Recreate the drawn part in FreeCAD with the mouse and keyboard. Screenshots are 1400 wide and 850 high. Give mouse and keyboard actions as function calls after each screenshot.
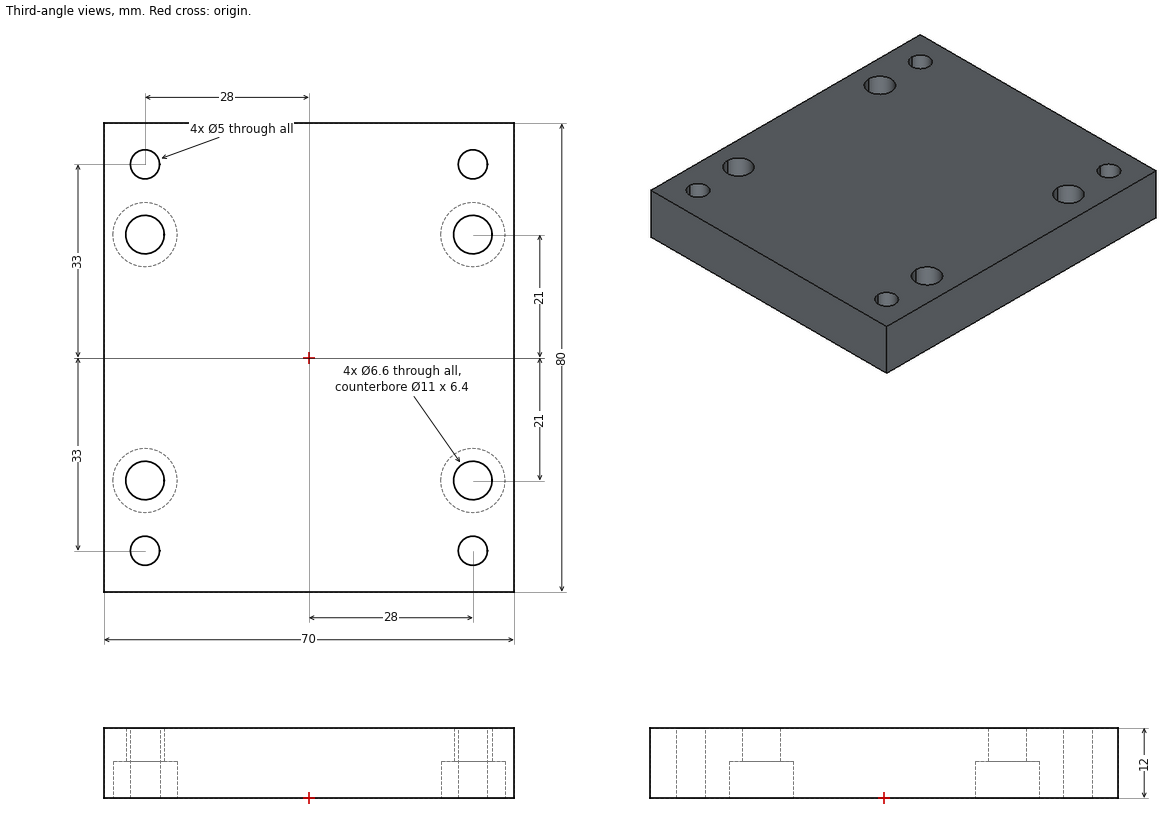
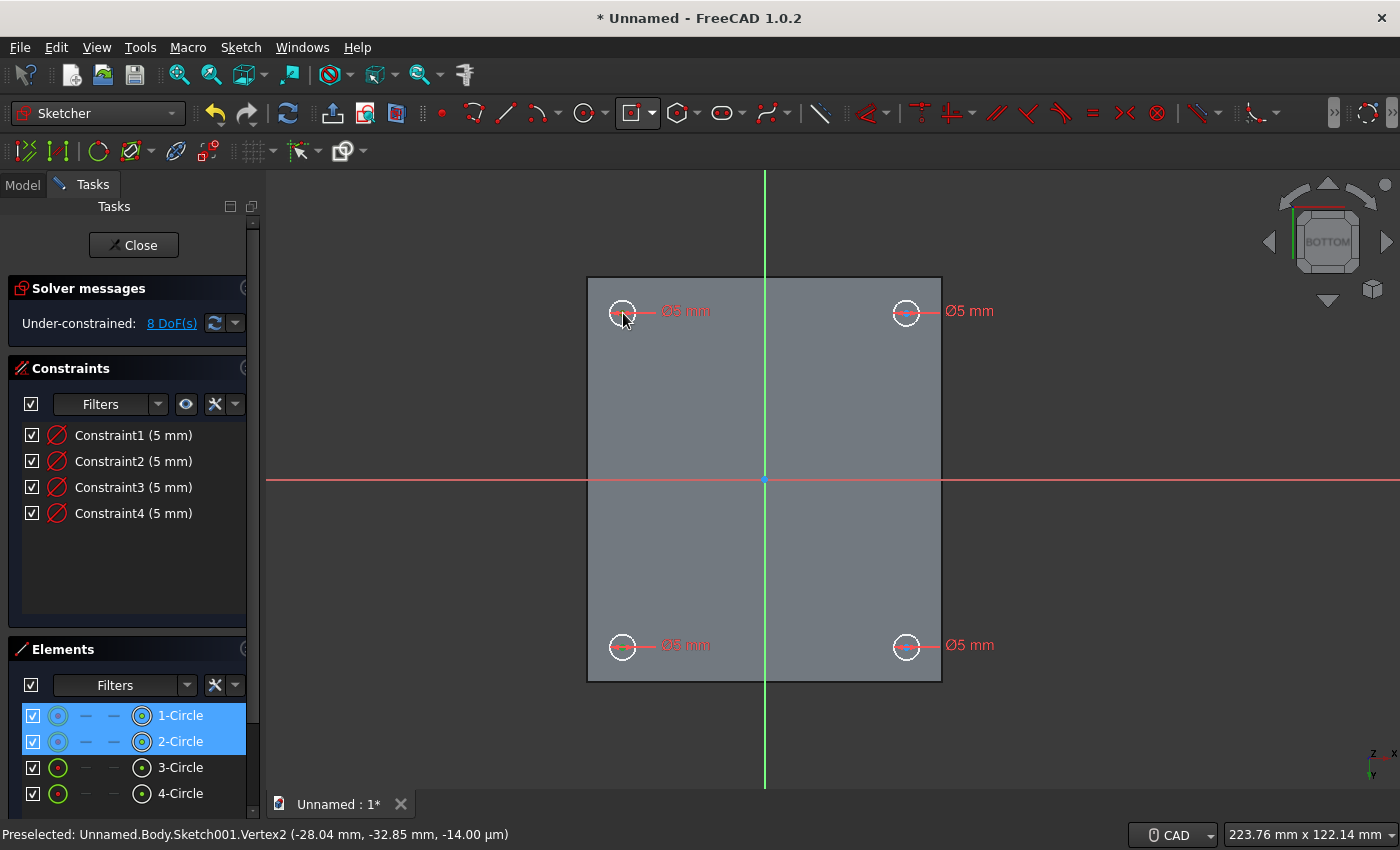
click(974, 114)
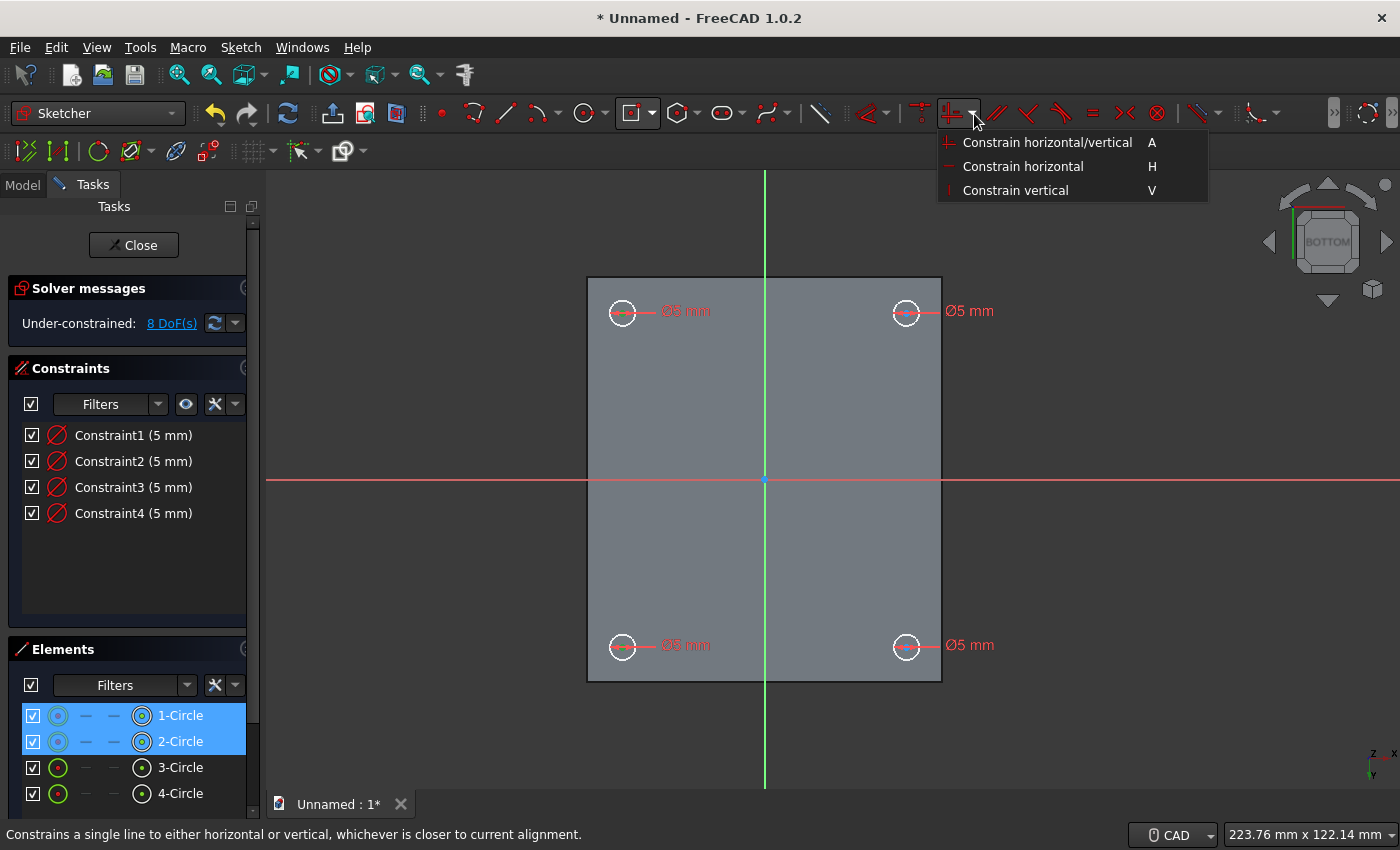
click(1073, 190)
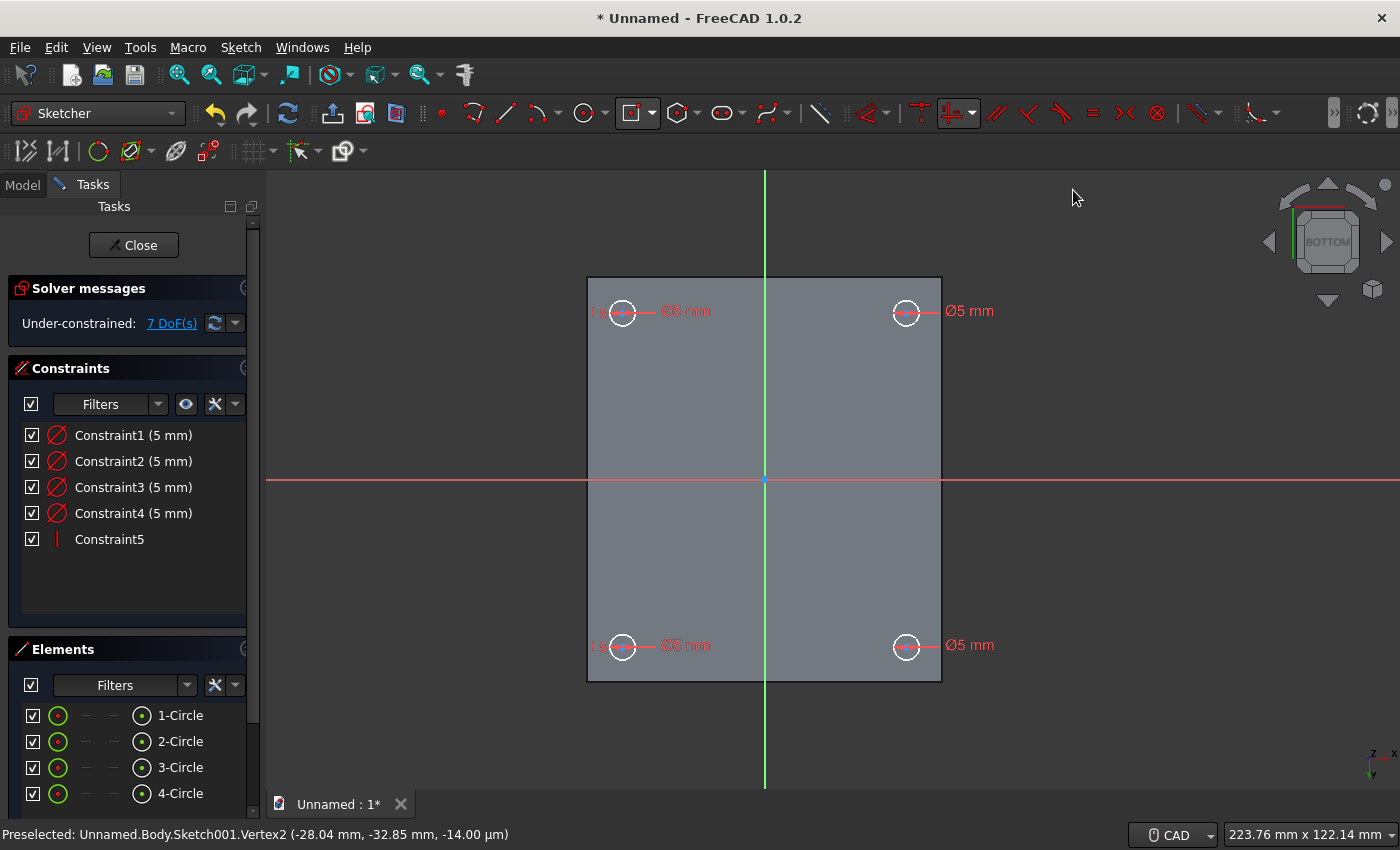
click(623, 313)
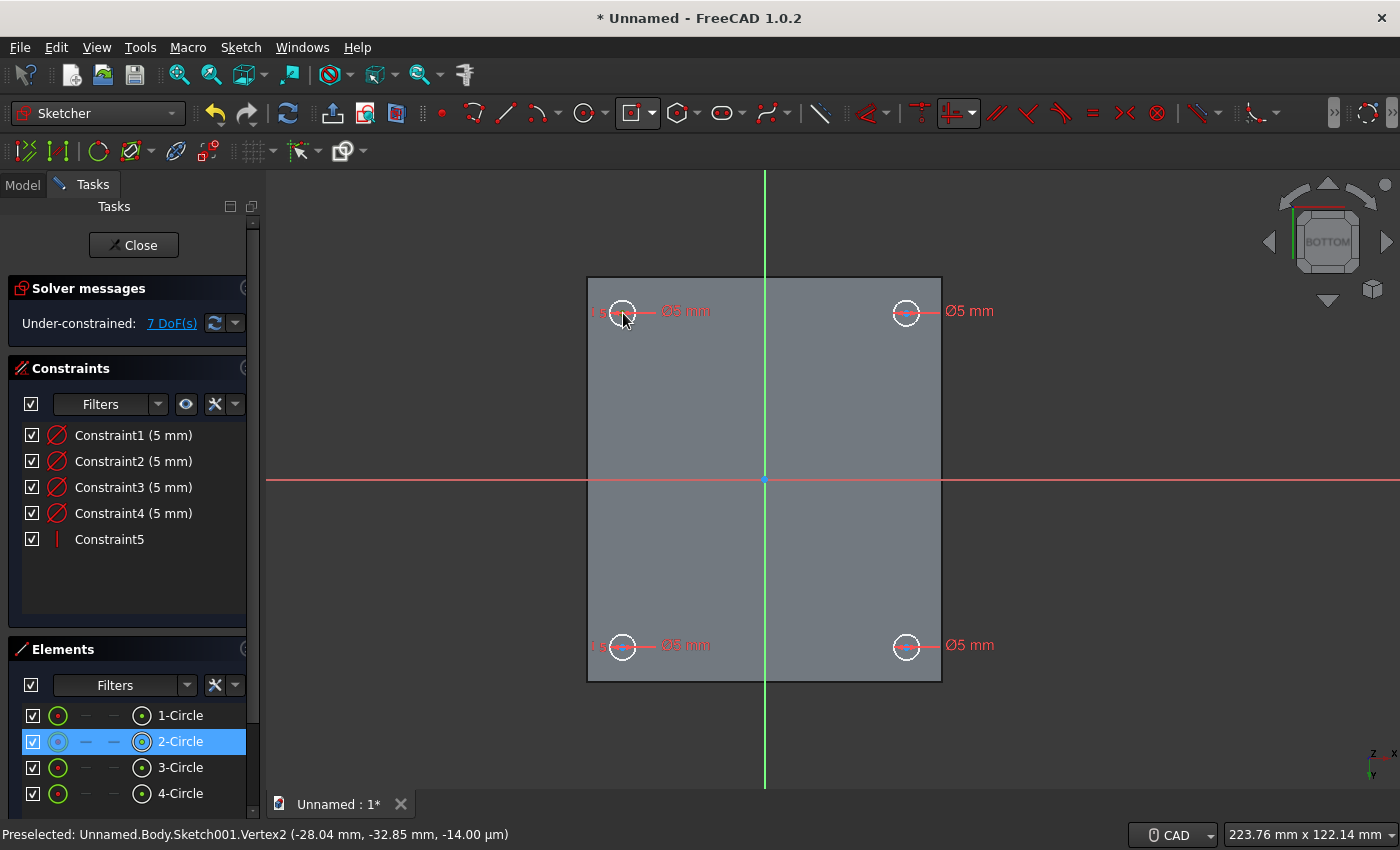
click(906, 313)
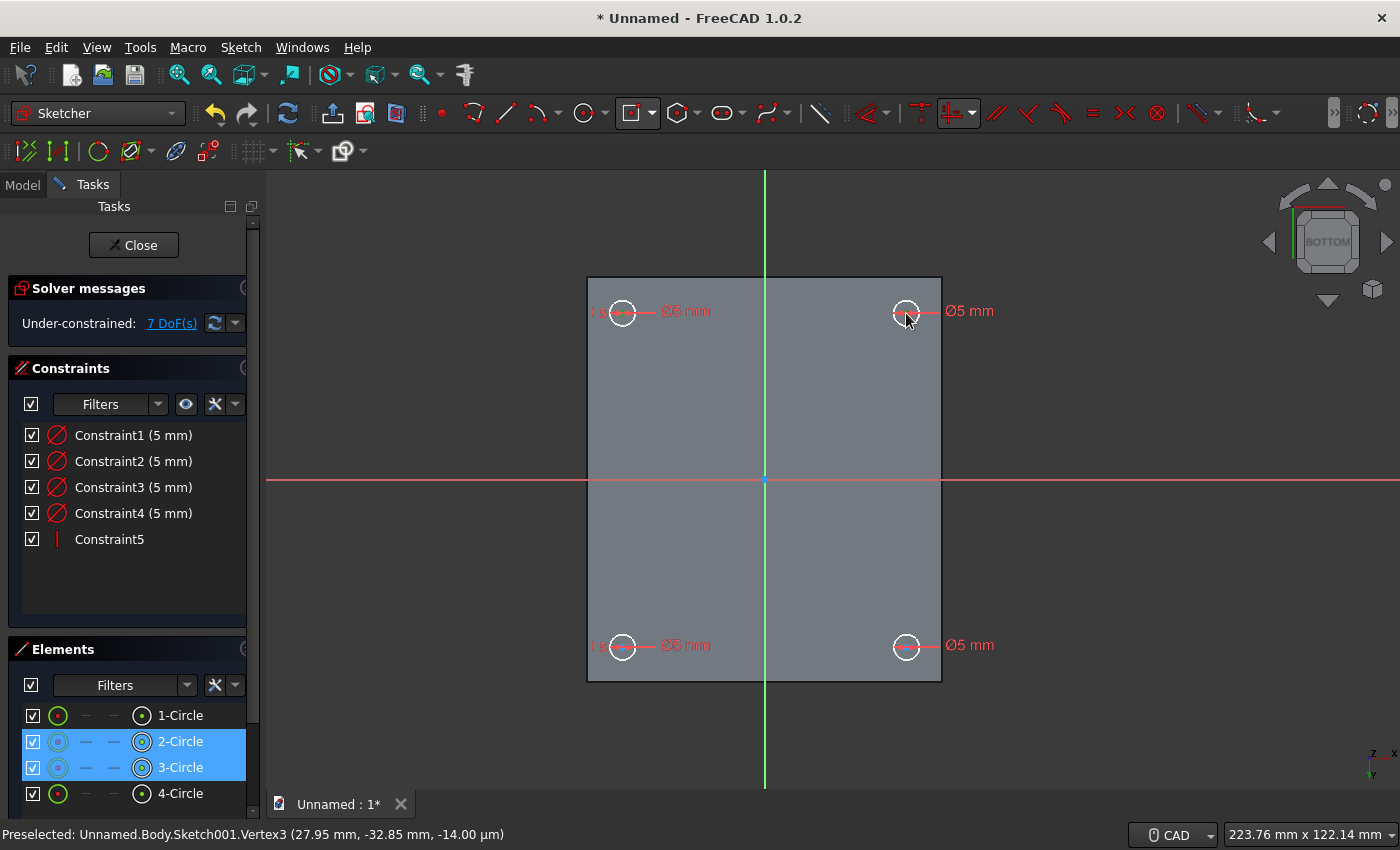
key(h)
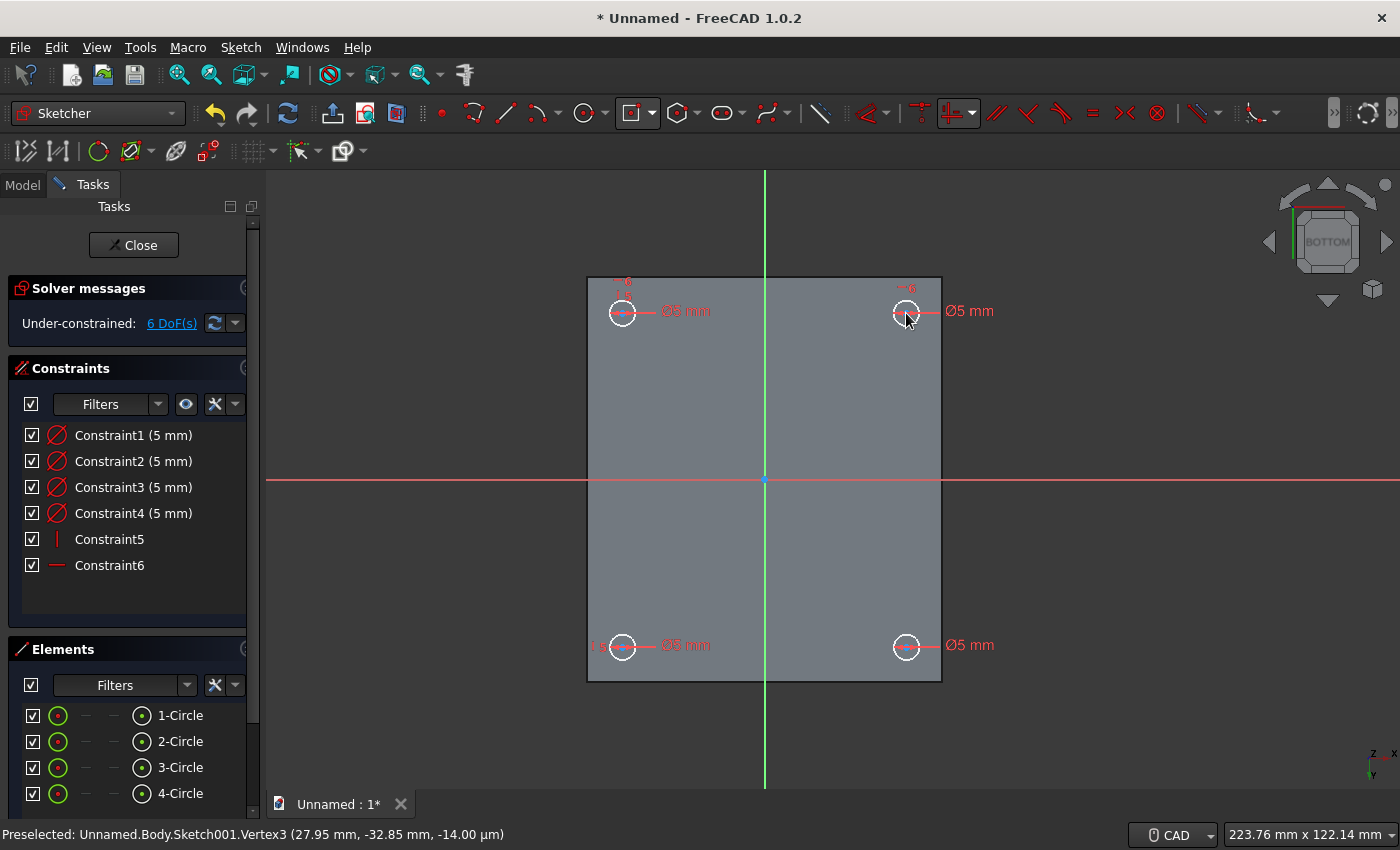
click(906, 313)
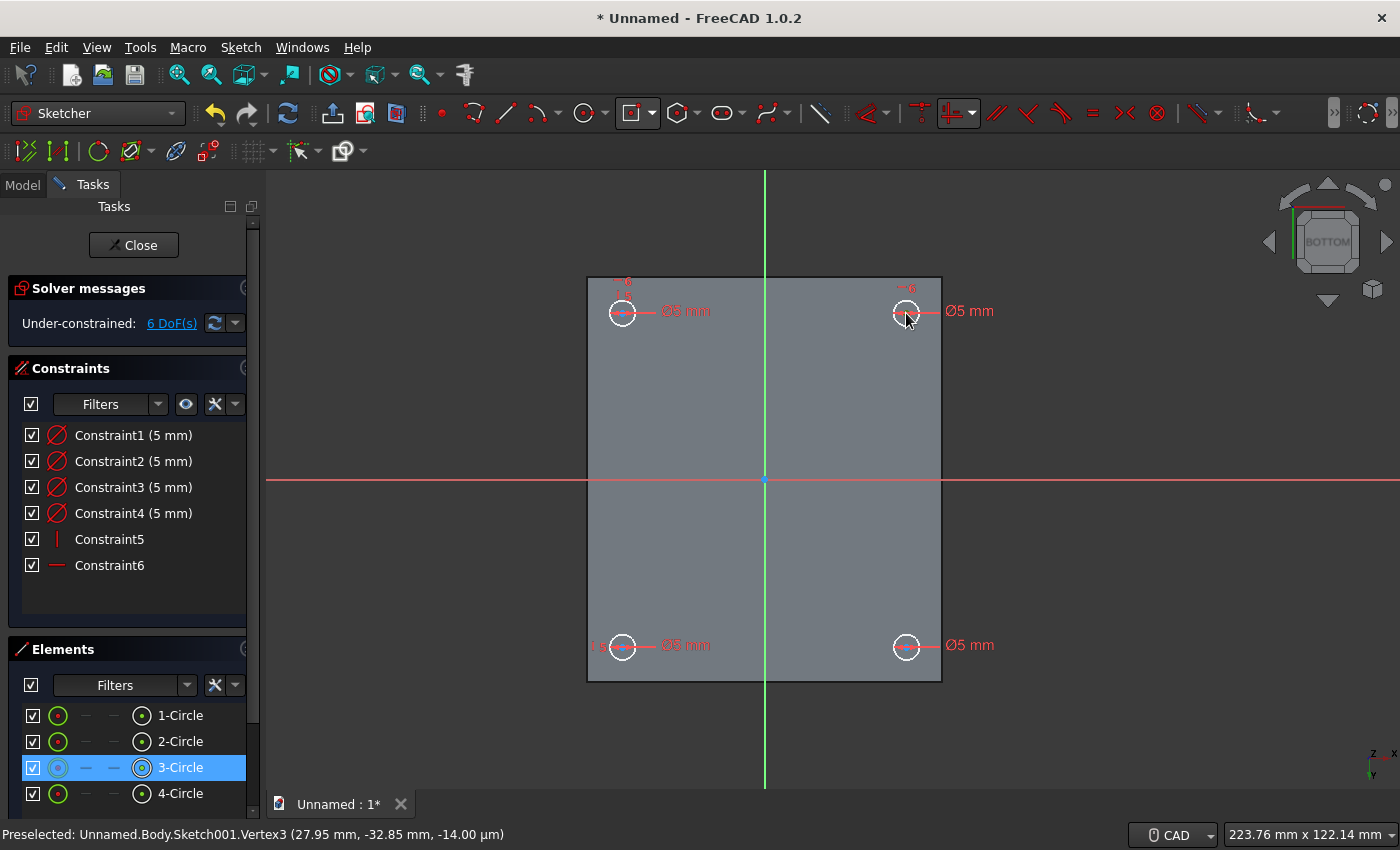
click(907, 647)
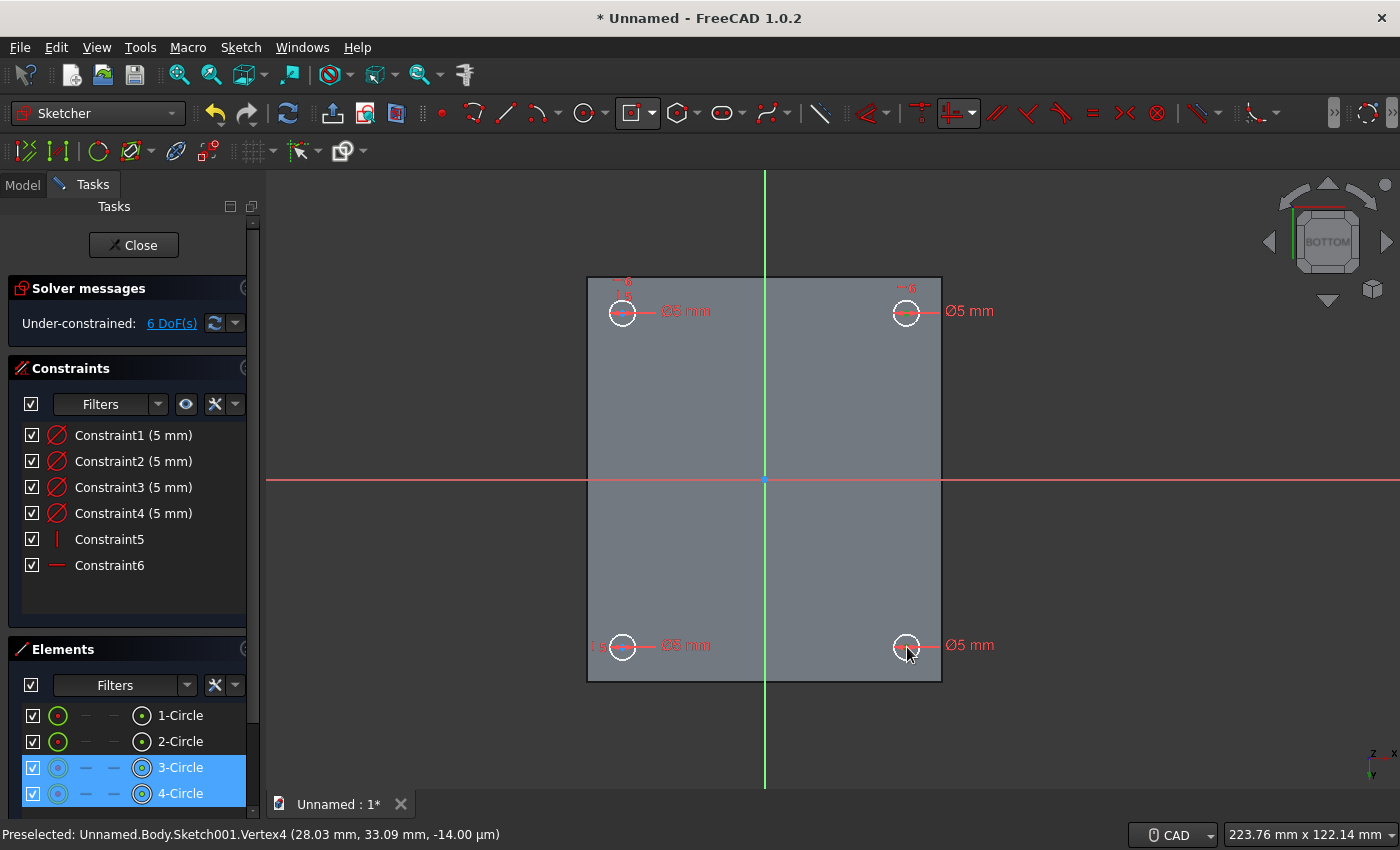
key(v)